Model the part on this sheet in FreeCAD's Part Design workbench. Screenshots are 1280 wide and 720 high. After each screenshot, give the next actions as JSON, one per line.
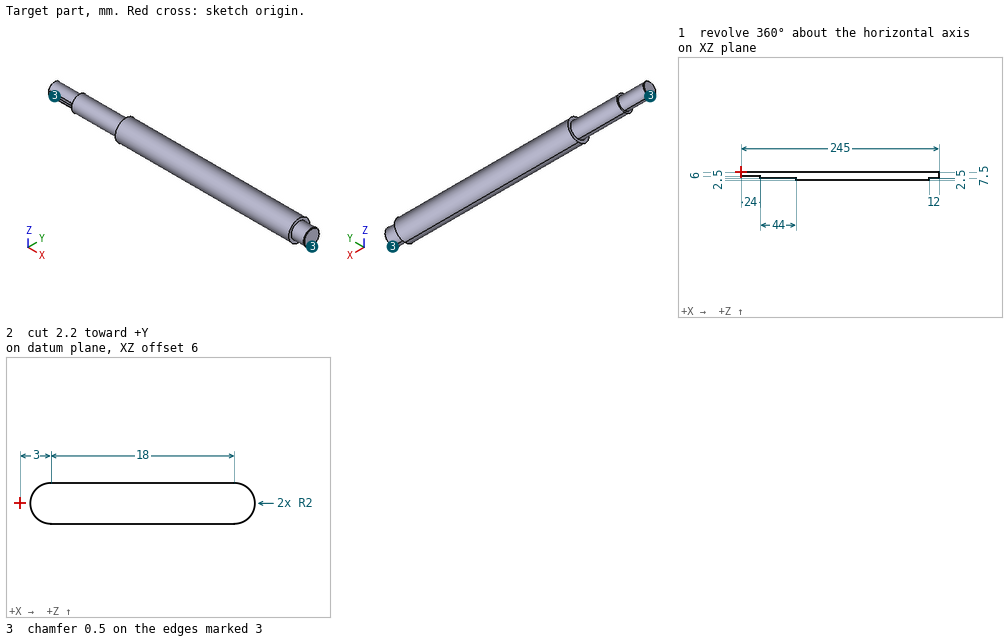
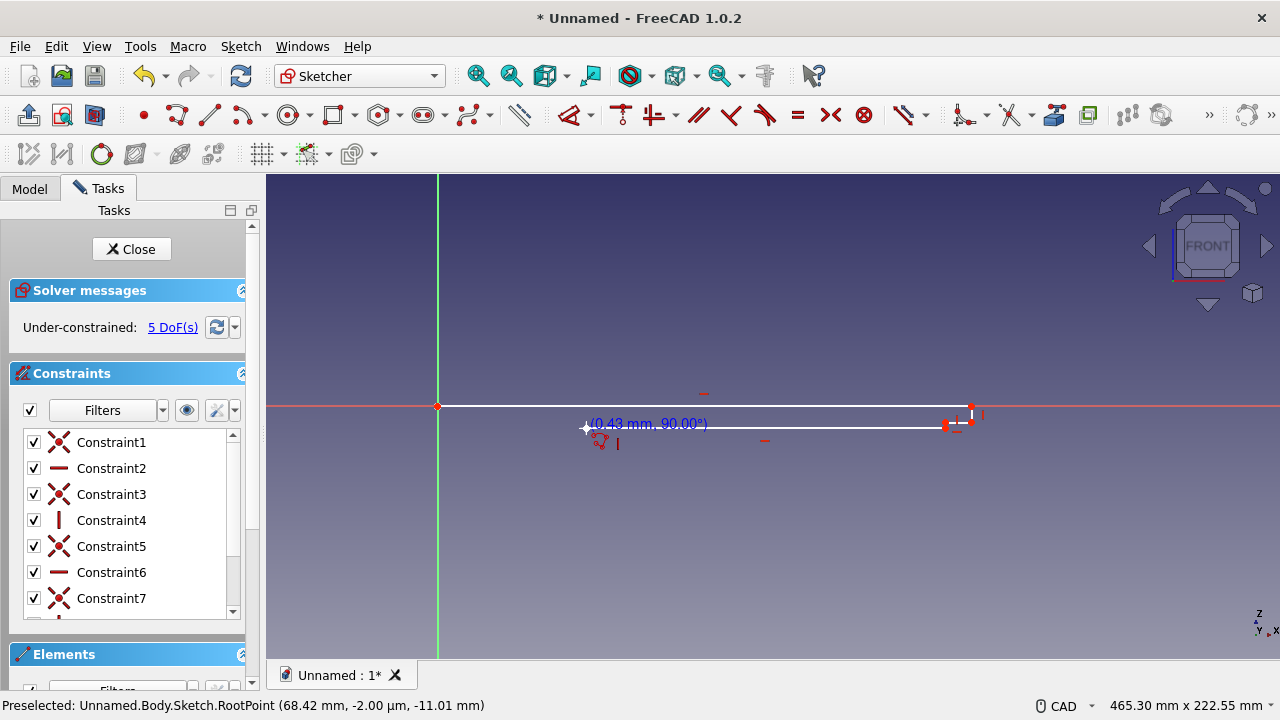
{"action": "scroll", "coordinate": [586, 422], "scroll_direction": "up", "scroll_amount": 6}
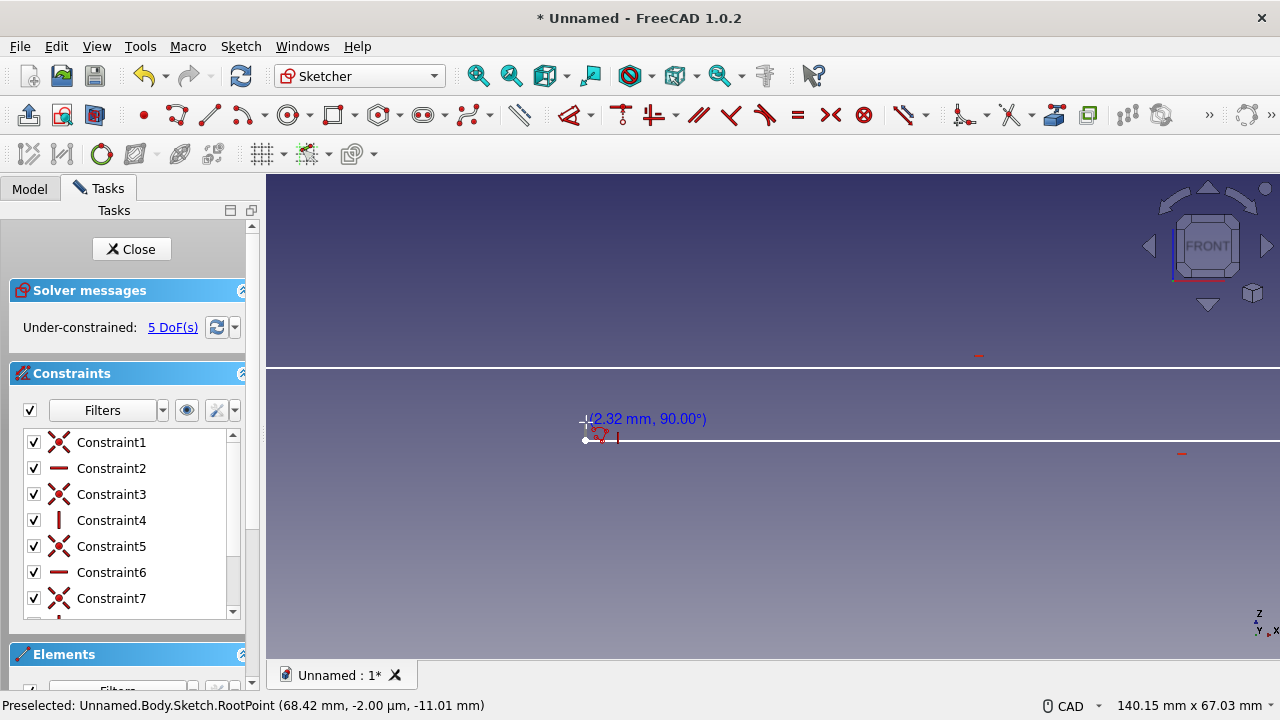
{"action": "left_click", "coordinate": [585, 422]}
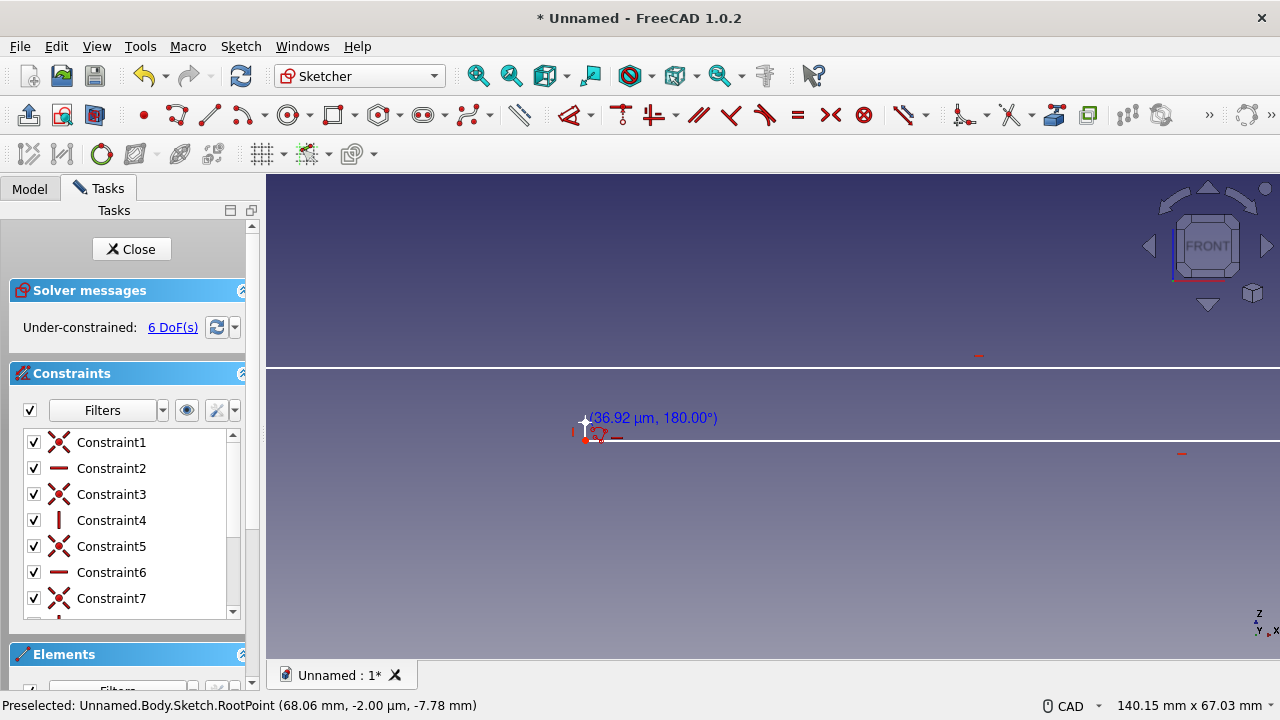
{"action": "scroll", "coordinate": [586, 422], "scroll_direction": "down", "scroll_amount": 6}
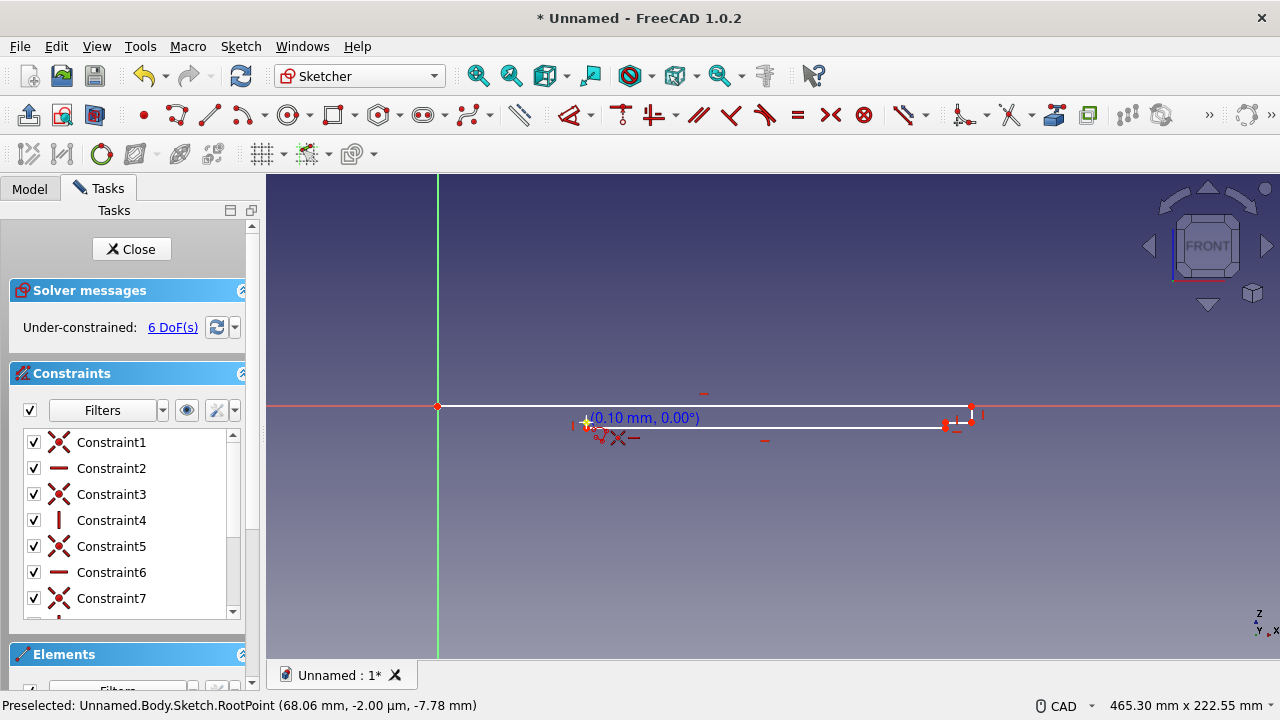
{"action": "left_click", "coordinate": [490, 422]}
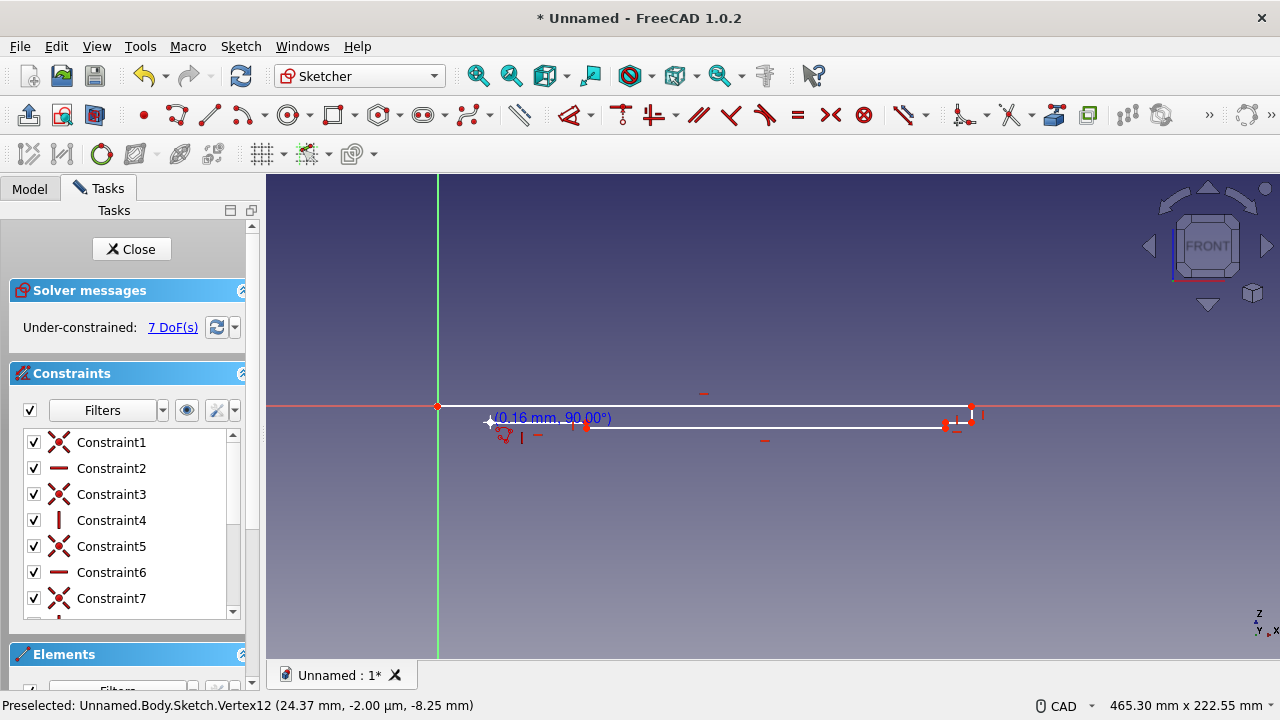
{"action": "scroll", "coordinate": [490, 419], "scroll_direction": "up", "scroll_amount": 8}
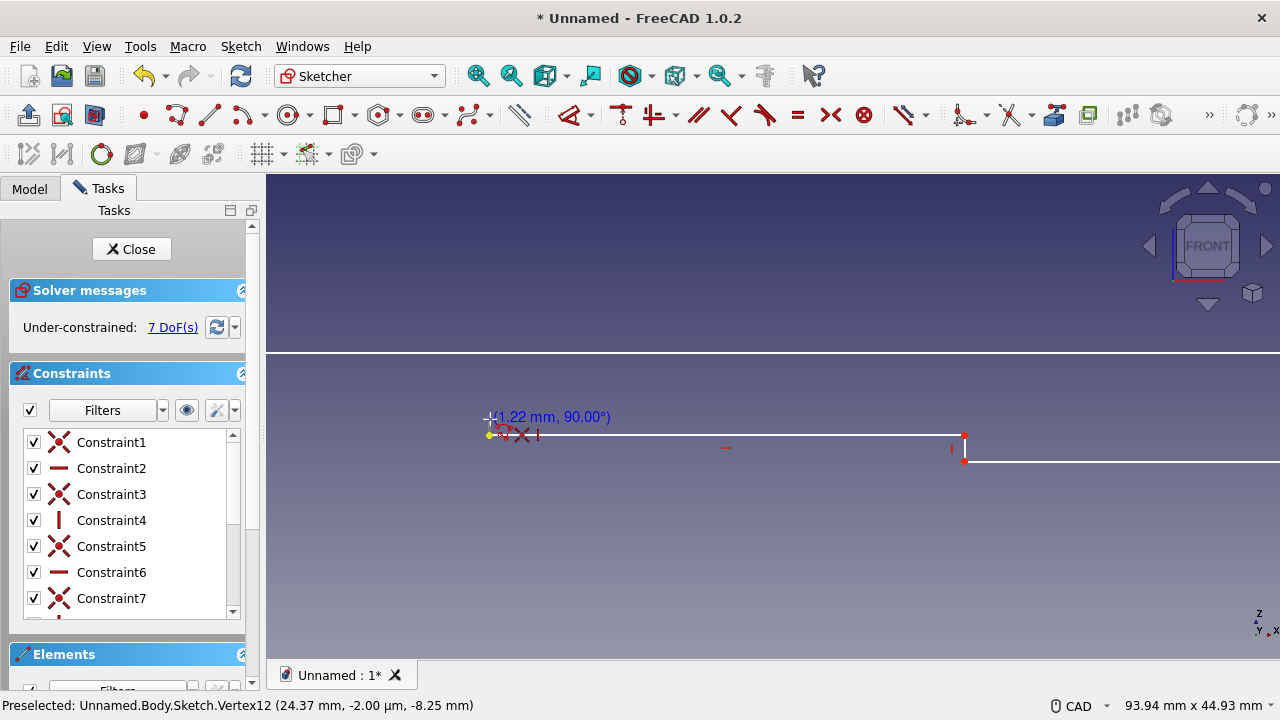
{"action": "left_click", "coordinate": [489, 417]}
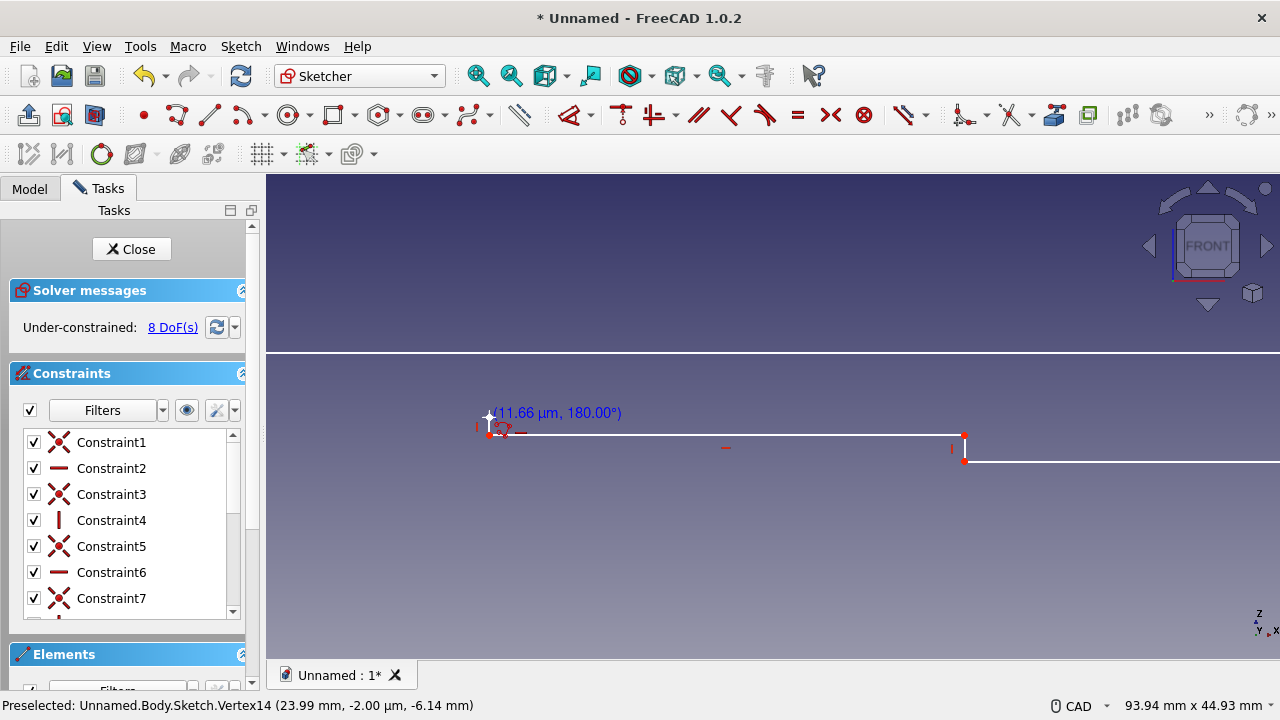
{"action": "scroll", "coordinate": [490, 419], "scroll_direction": "down", "scroll_amount": 8}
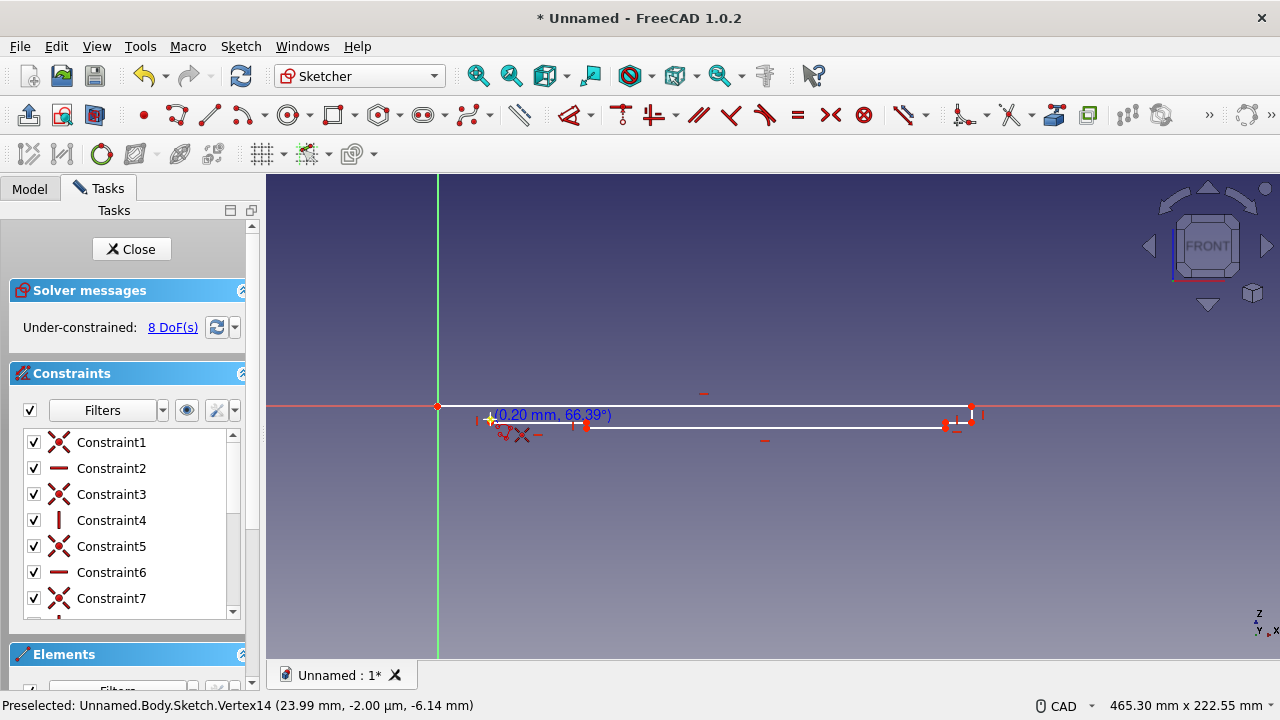
{"action": "left_click", "coordinate": [447, 419]}
{"action": "left_click", "coordinate": [438, 406]}
{"action": "key", "text": "Escape"}
{"action": "key", "text": "Escape"}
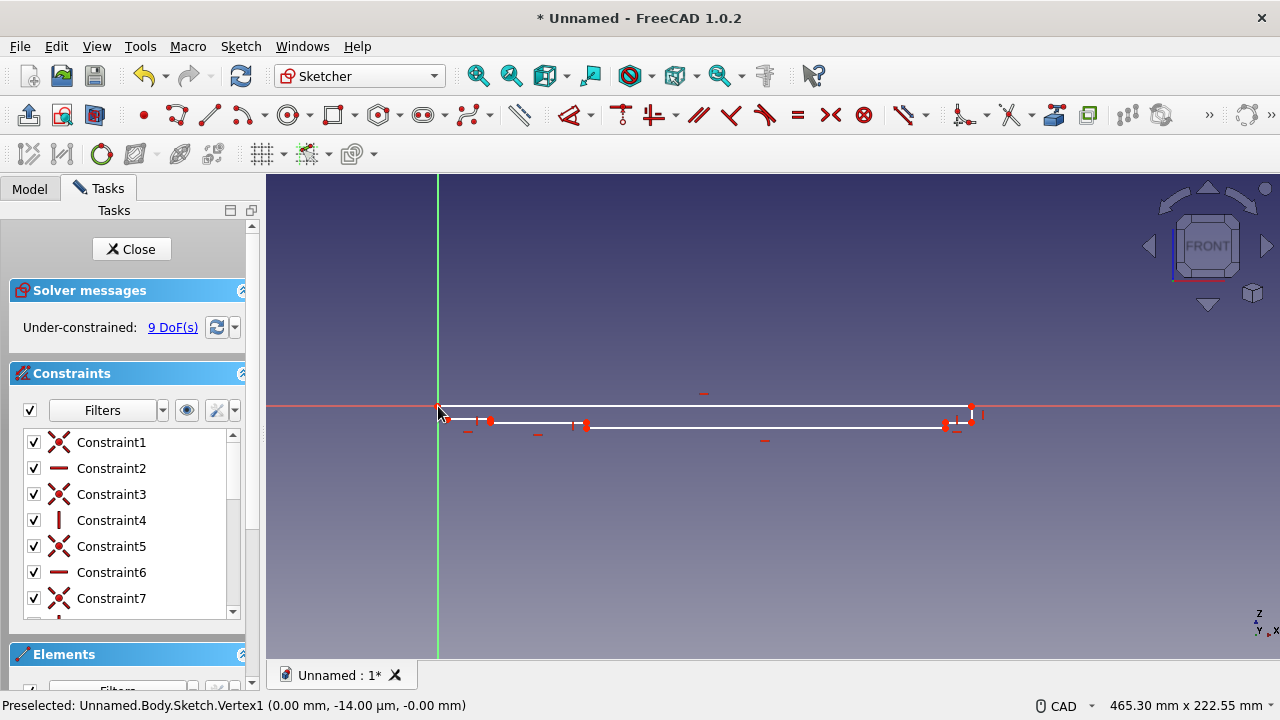
{"action": "scroll", "coordinate": [443, 414], "scroll_direction": "up", "scroll_amount": 5}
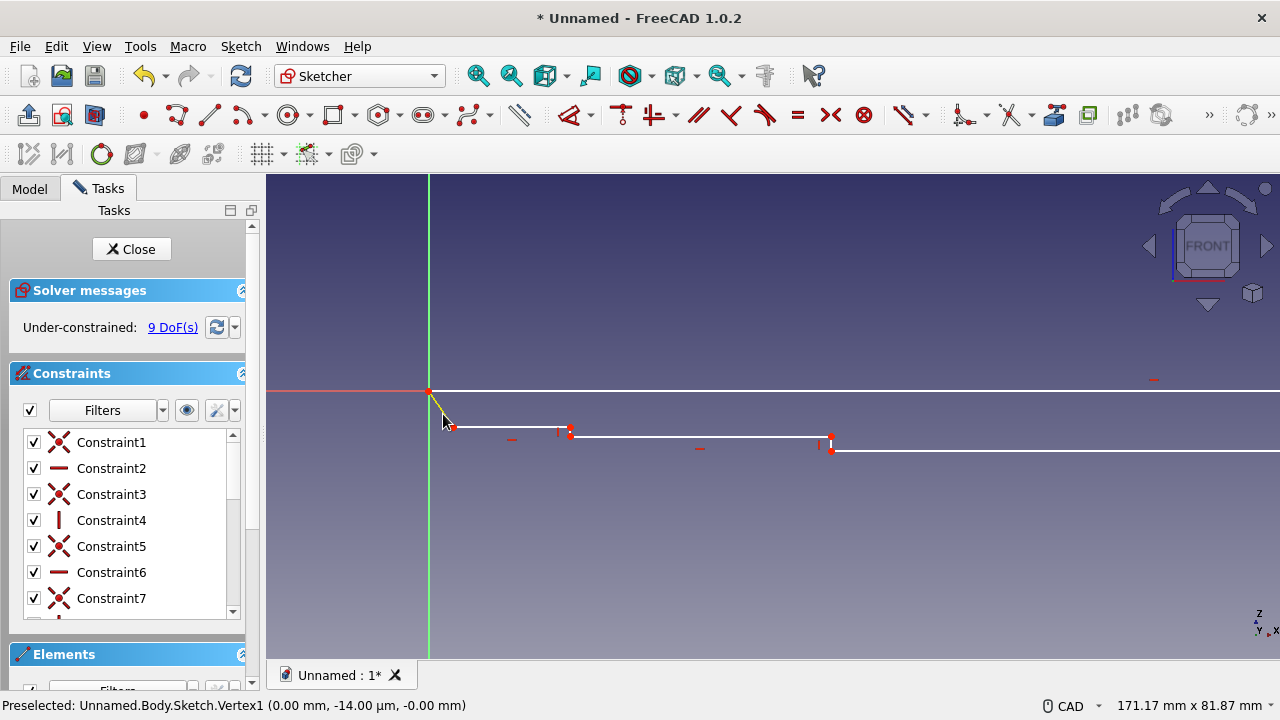
{"action": "left_click", "coordinate": [444, 413]}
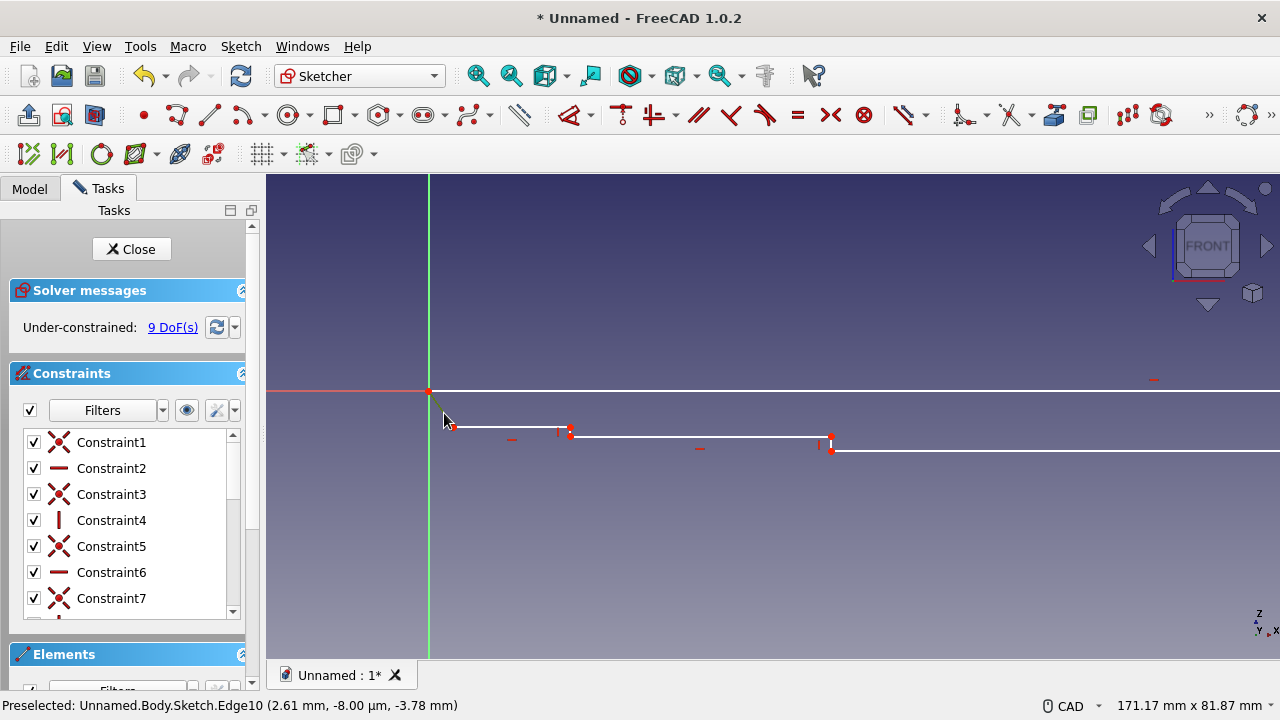
{"action": "left_click", "coordinate": [676, 116]}